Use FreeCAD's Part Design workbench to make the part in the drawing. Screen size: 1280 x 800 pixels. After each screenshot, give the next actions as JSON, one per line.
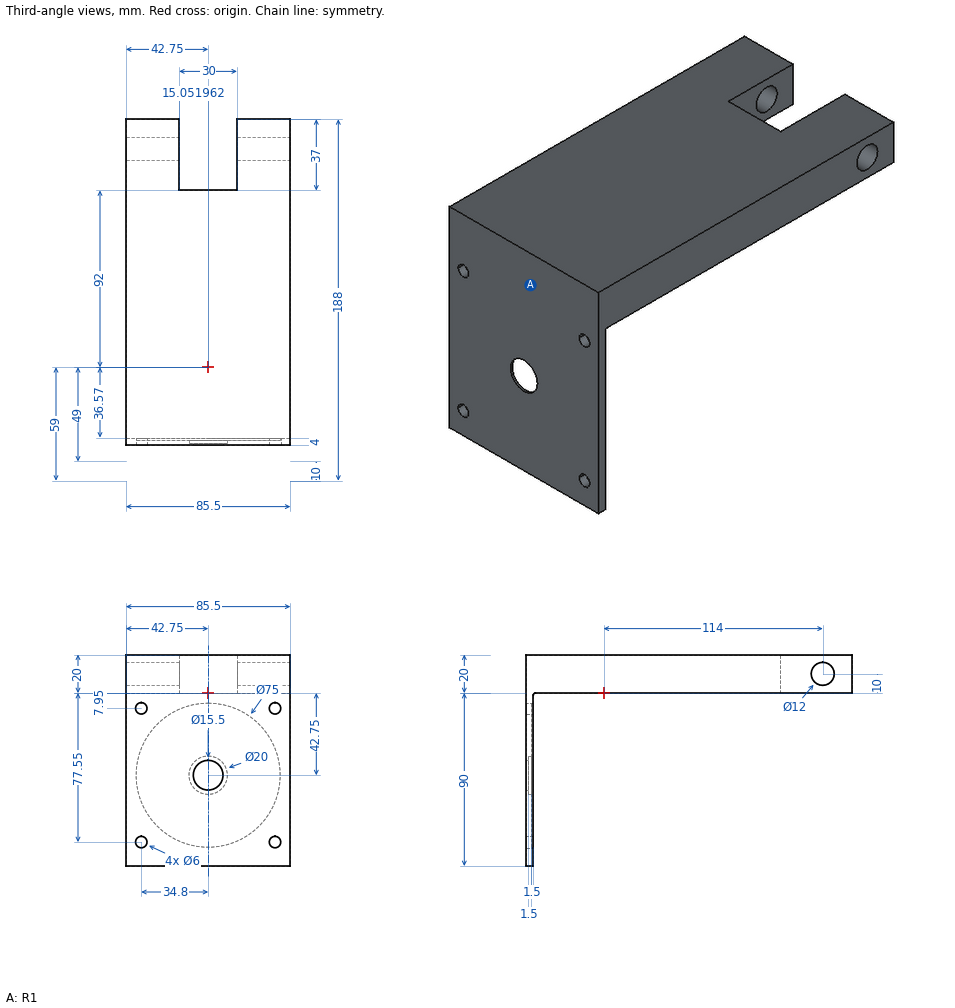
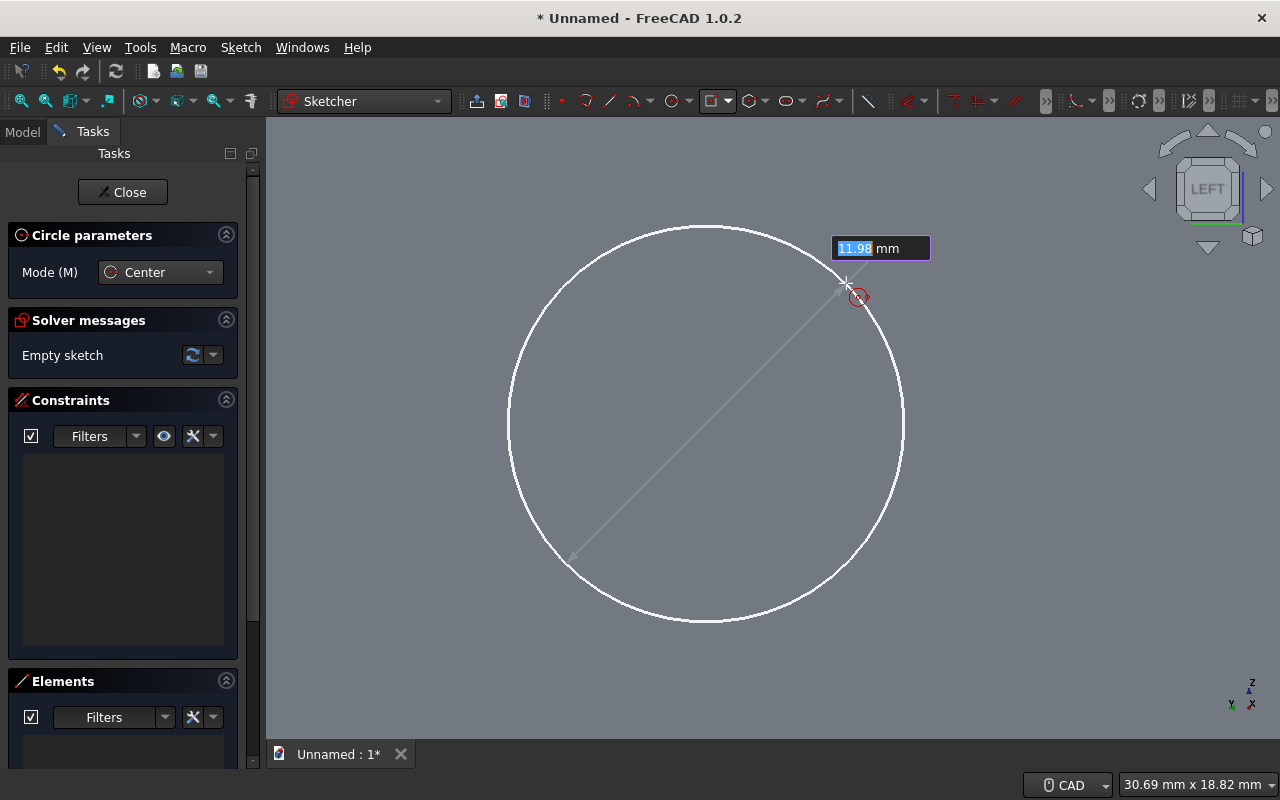
{"action": "type", "text": "12"}
{"action": "key", "text": "Return"}
{"action": "key", "text": "Escape"}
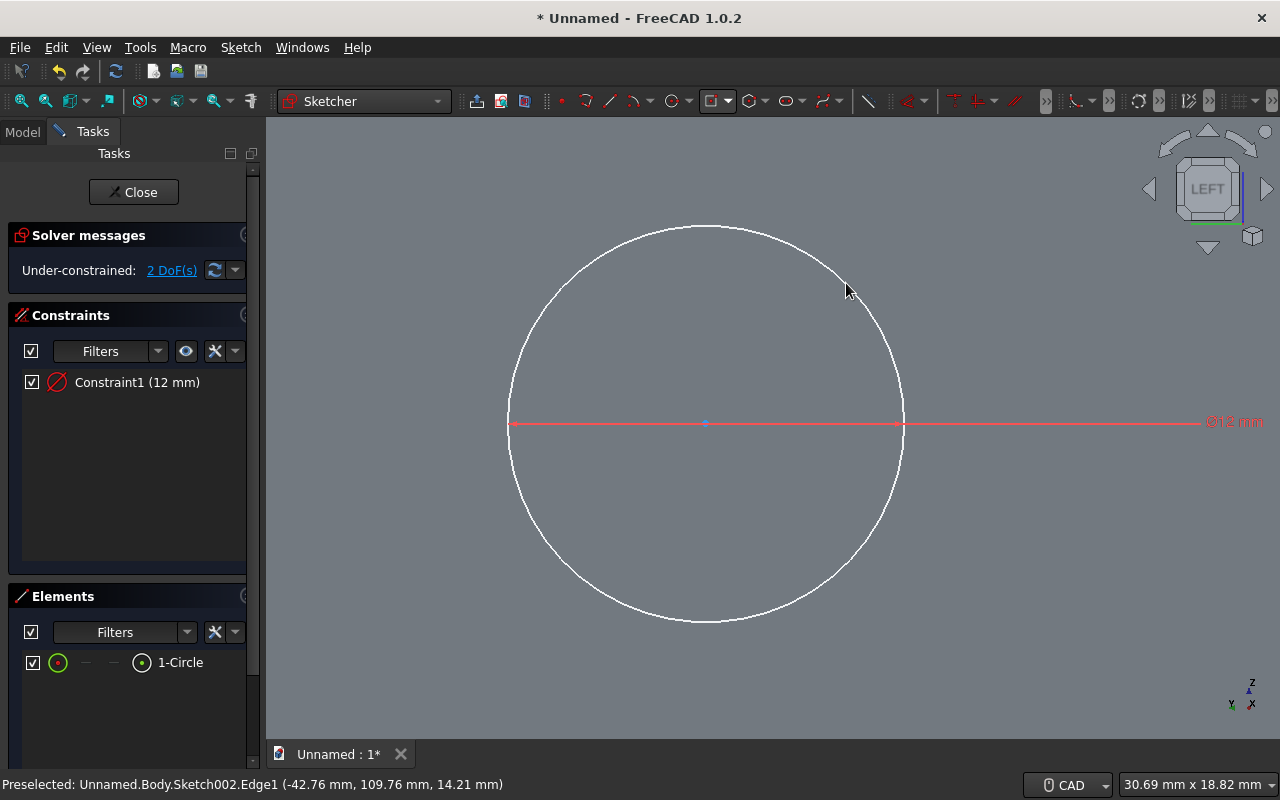
{"action": "left_click", "coordinate": [908, 102]}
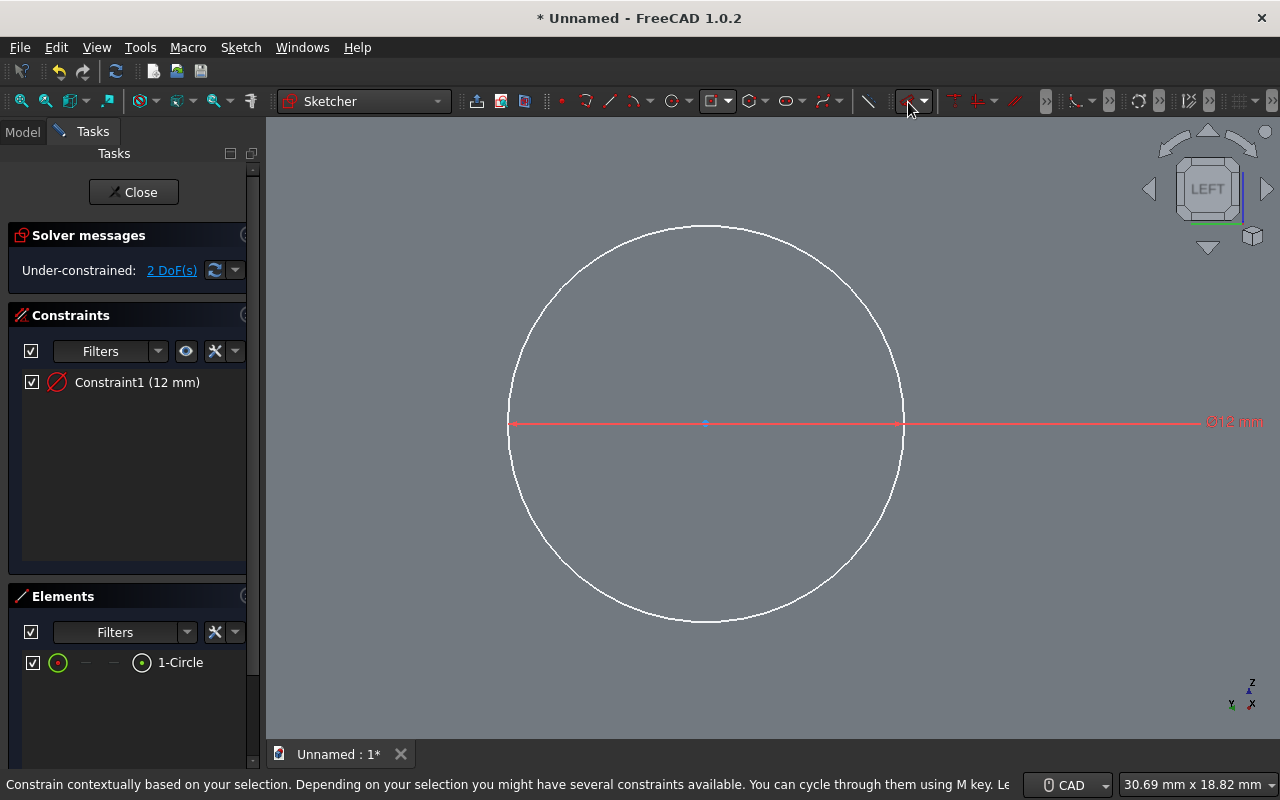
{"action": "left_click", "coordinate": [706, 424]}
{"action": "left_click", "coordinate": [672, 567]}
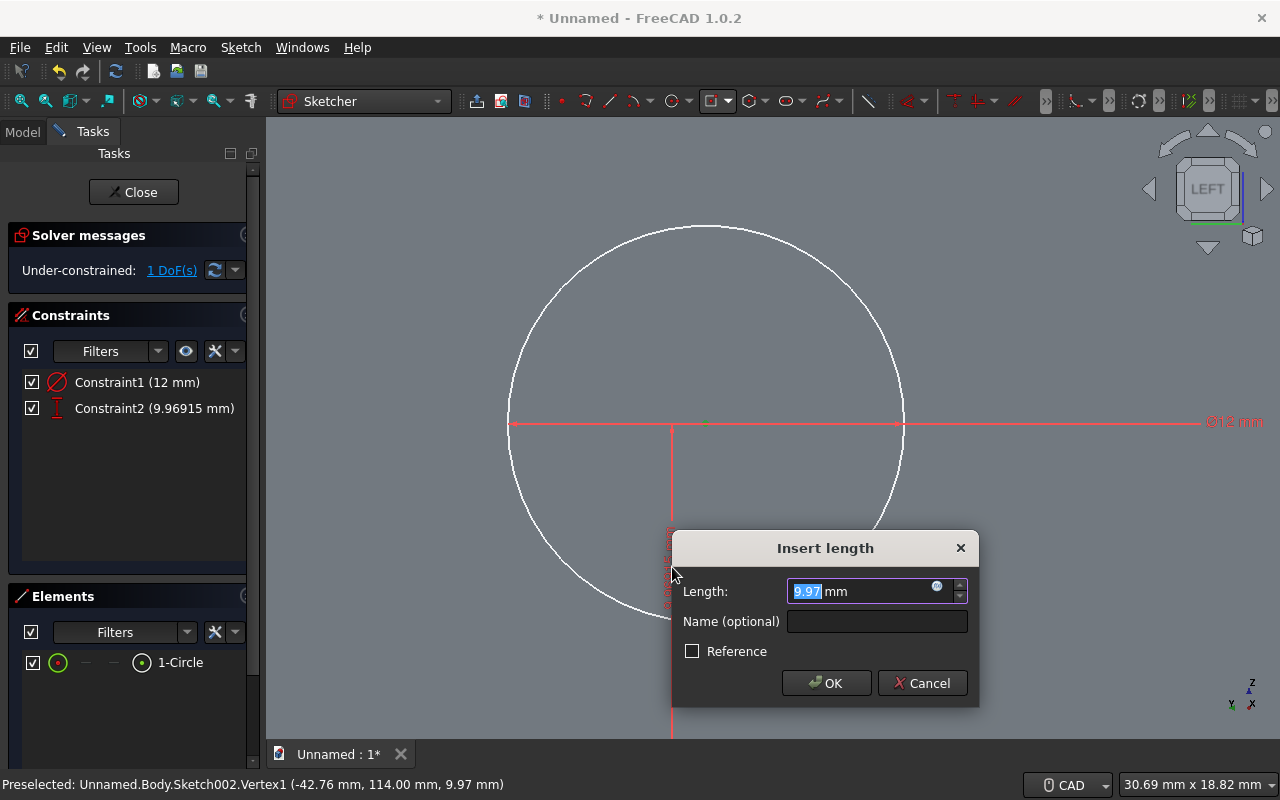
{"action": "type", "text": "10"}
{"action": "key", "text": "Return"}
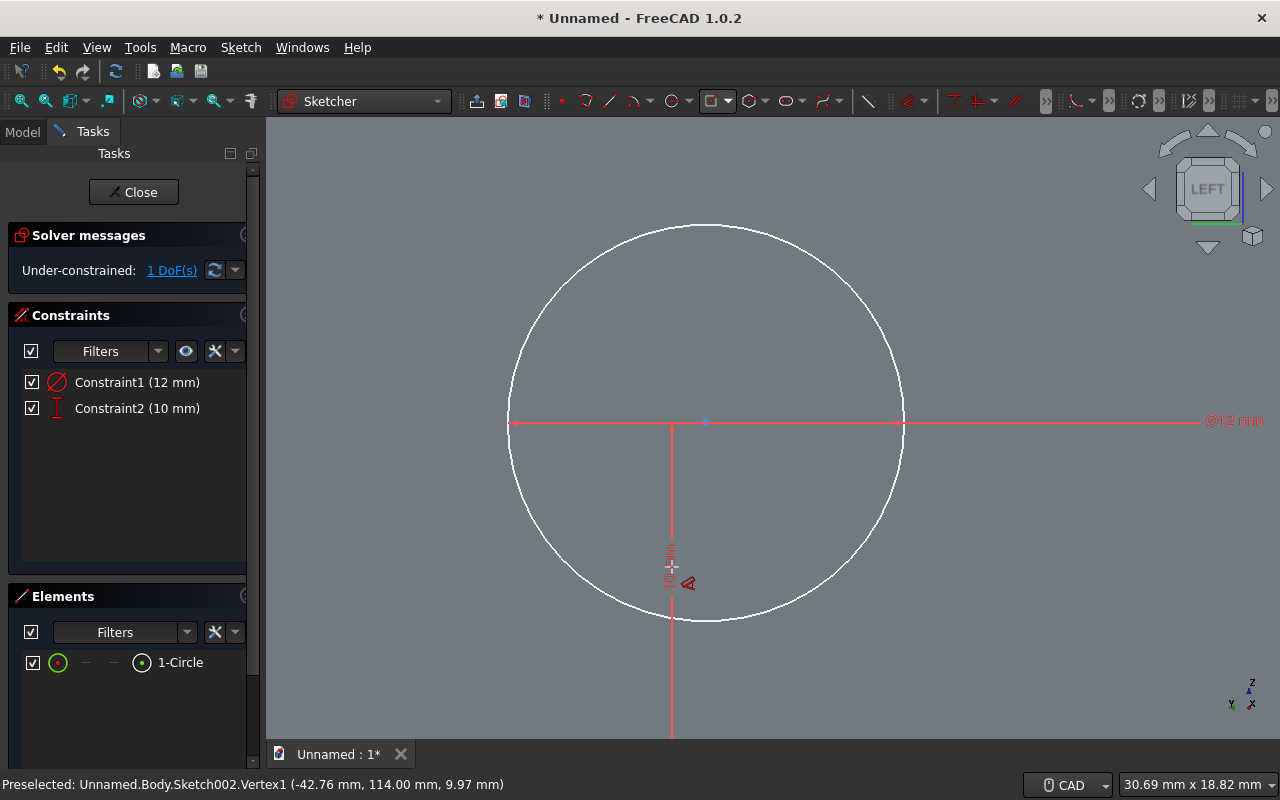
{"action": "left_click", "coordinate": [706, 423]}
{"action": "left_click", "coordinate": [816, 389]}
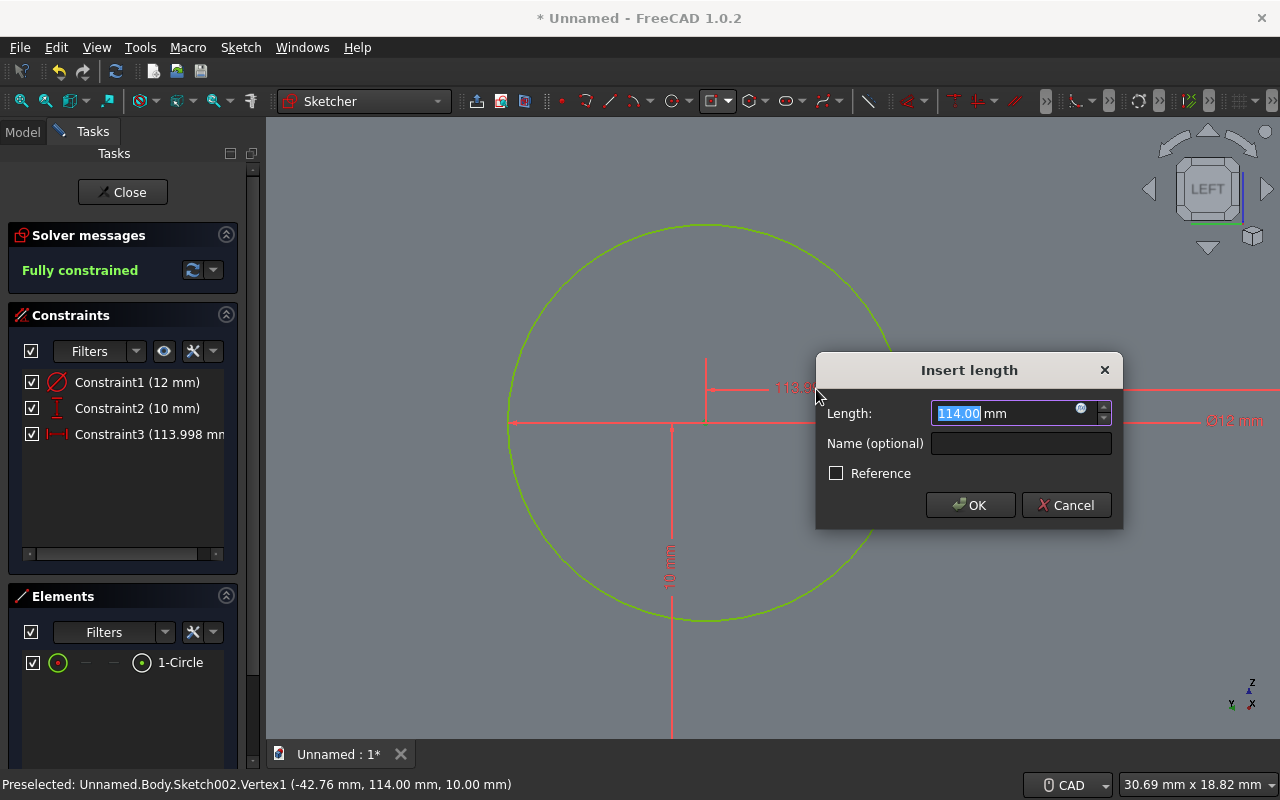
{"action": "type", "text": "114"}
{"action": "key", "text": "Return"}
{"action": "key", "text": "Escape"}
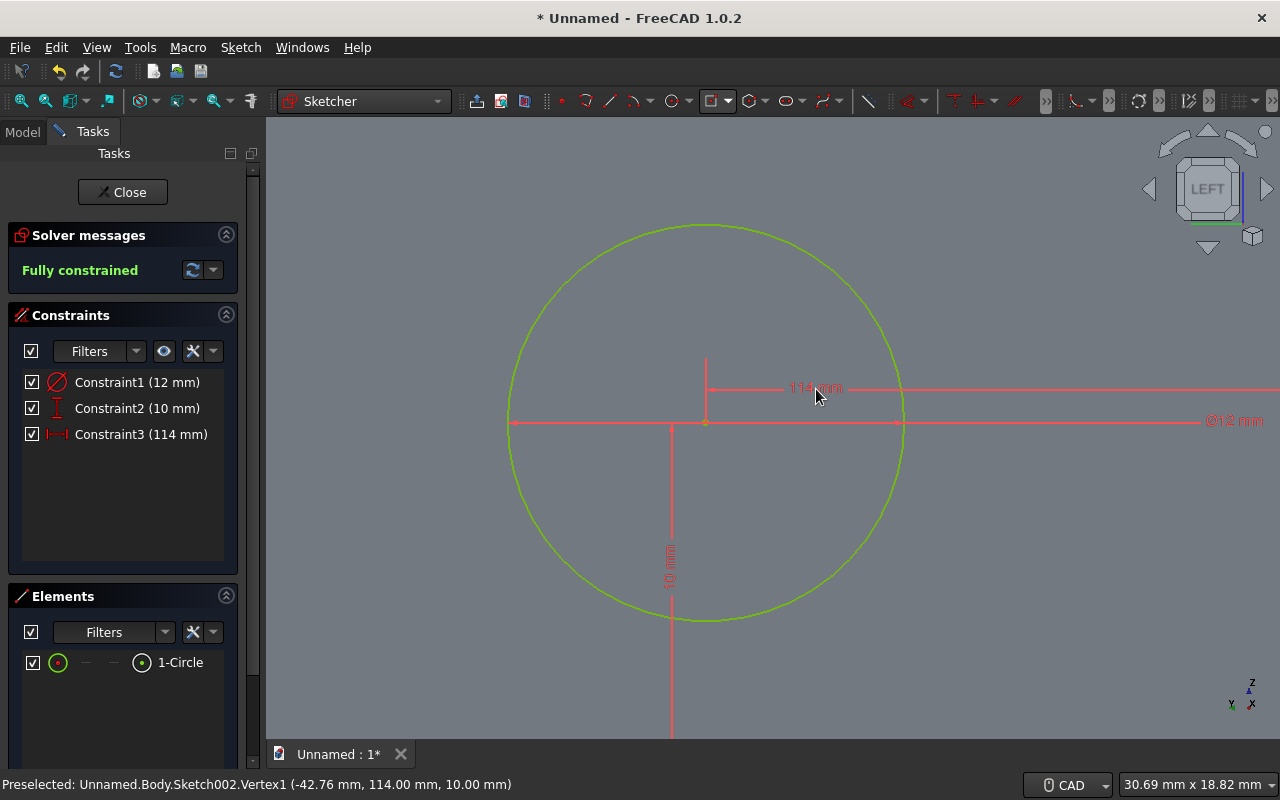
{"action": "left_click", "coordinate": [123, 192]}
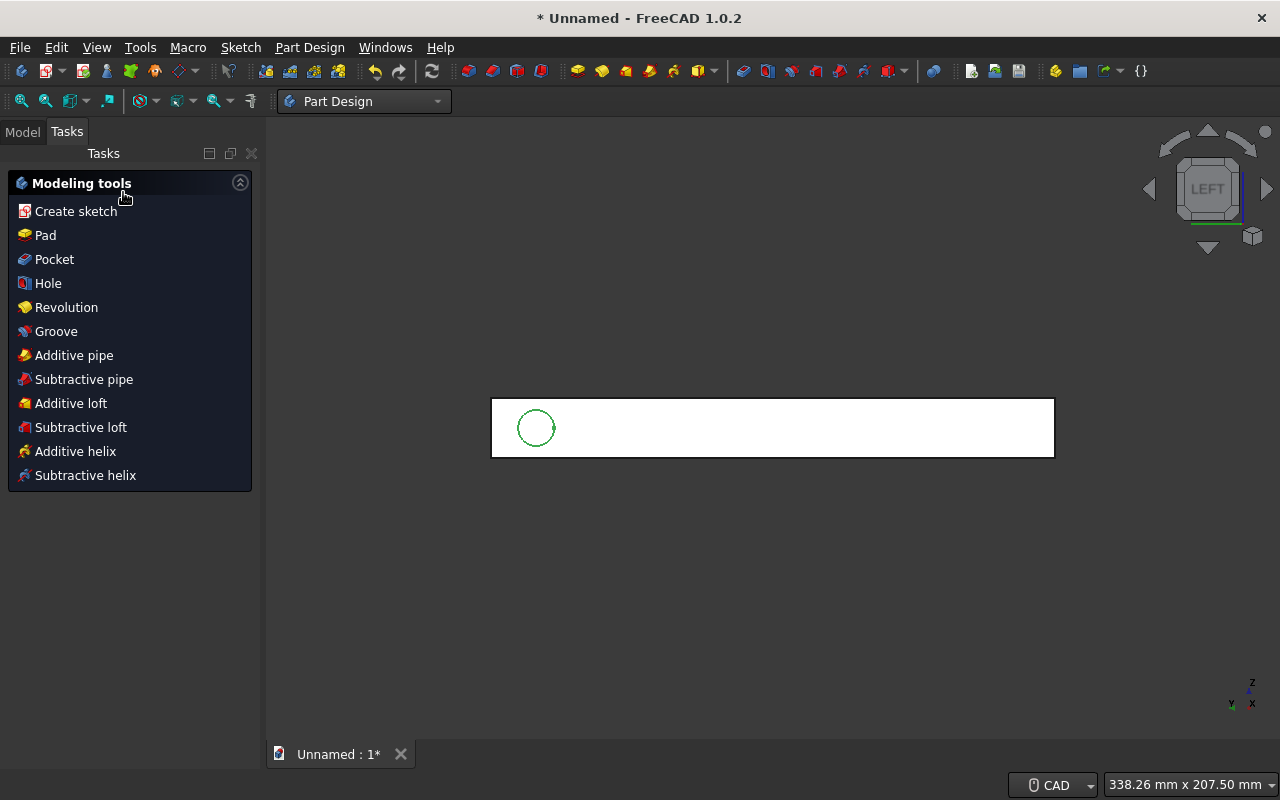
{"action": "left_click", "coordinate": [744, 72]}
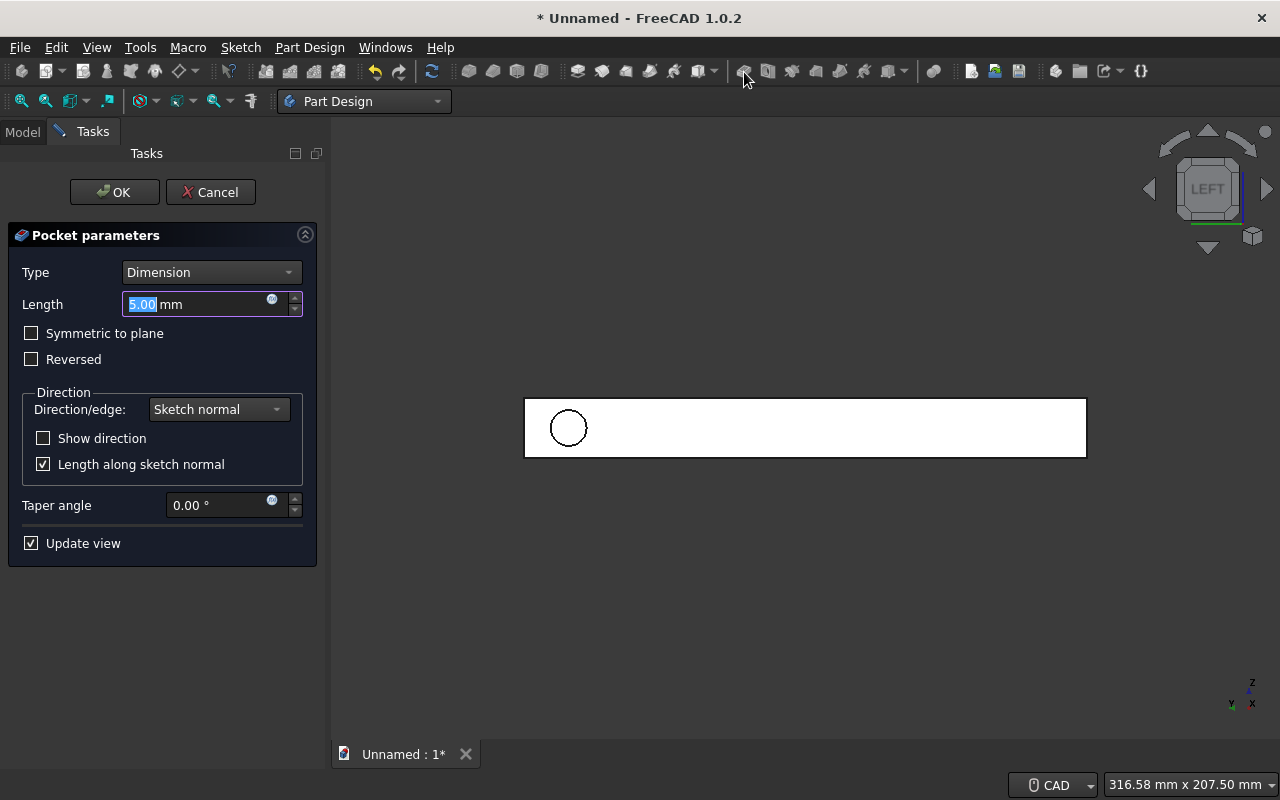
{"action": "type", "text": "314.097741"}
{"action": "key", "text": "Tab"}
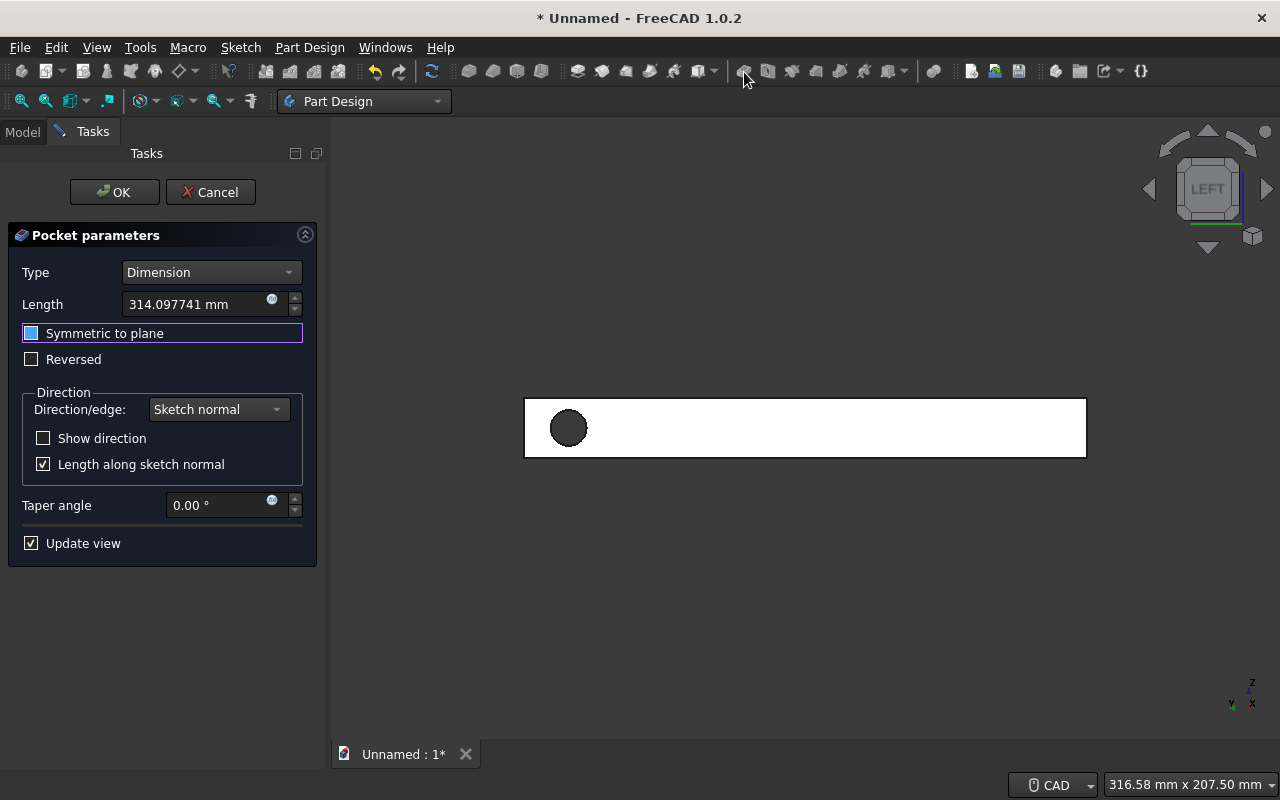
{"action": "left_click", "coordinate": [30, 333]}